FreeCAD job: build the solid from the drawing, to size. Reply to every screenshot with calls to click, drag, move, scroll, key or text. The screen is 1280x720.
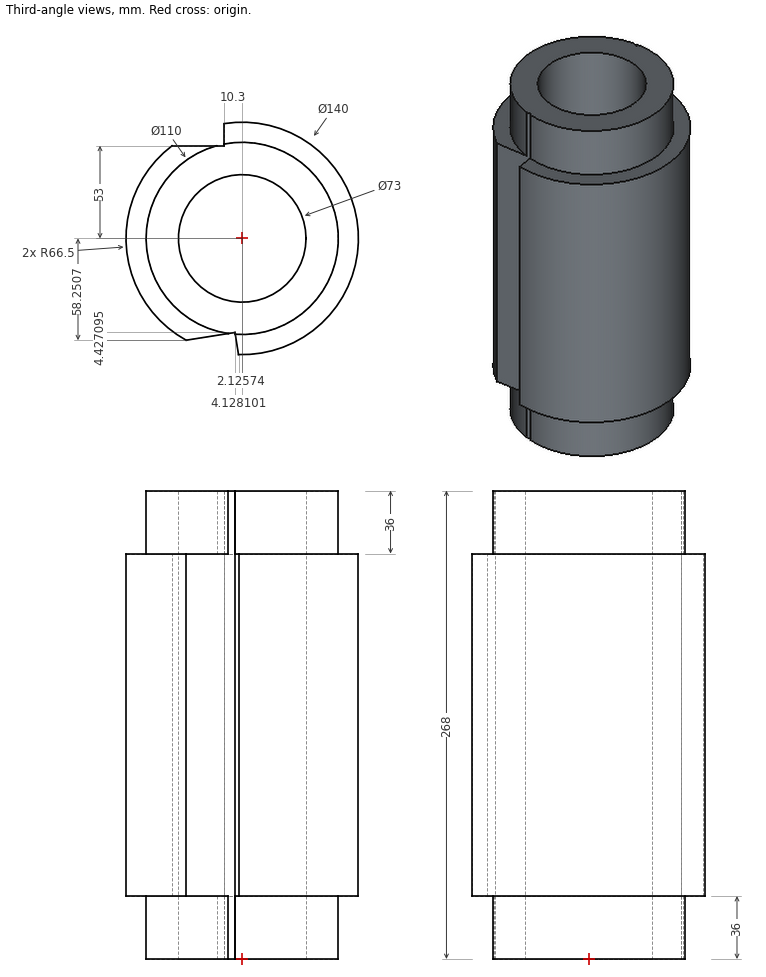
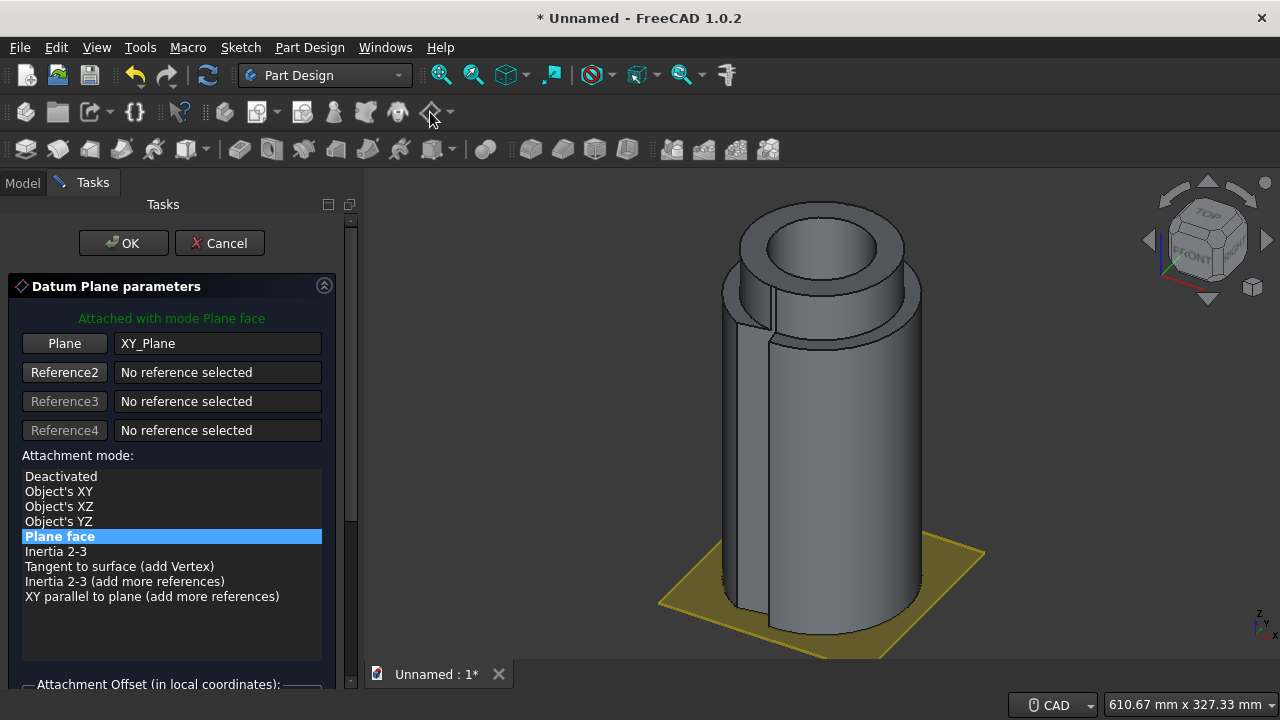
scroll(351, 451, down, 3)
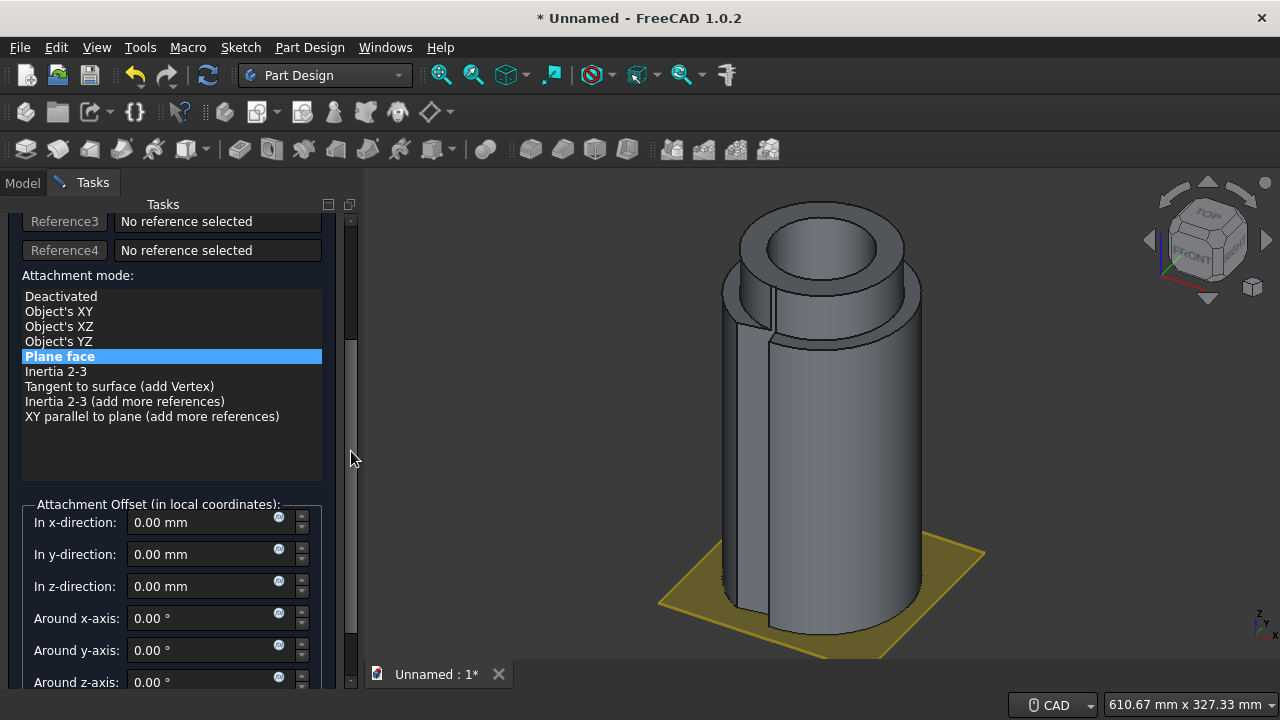
triple_click(210, 586)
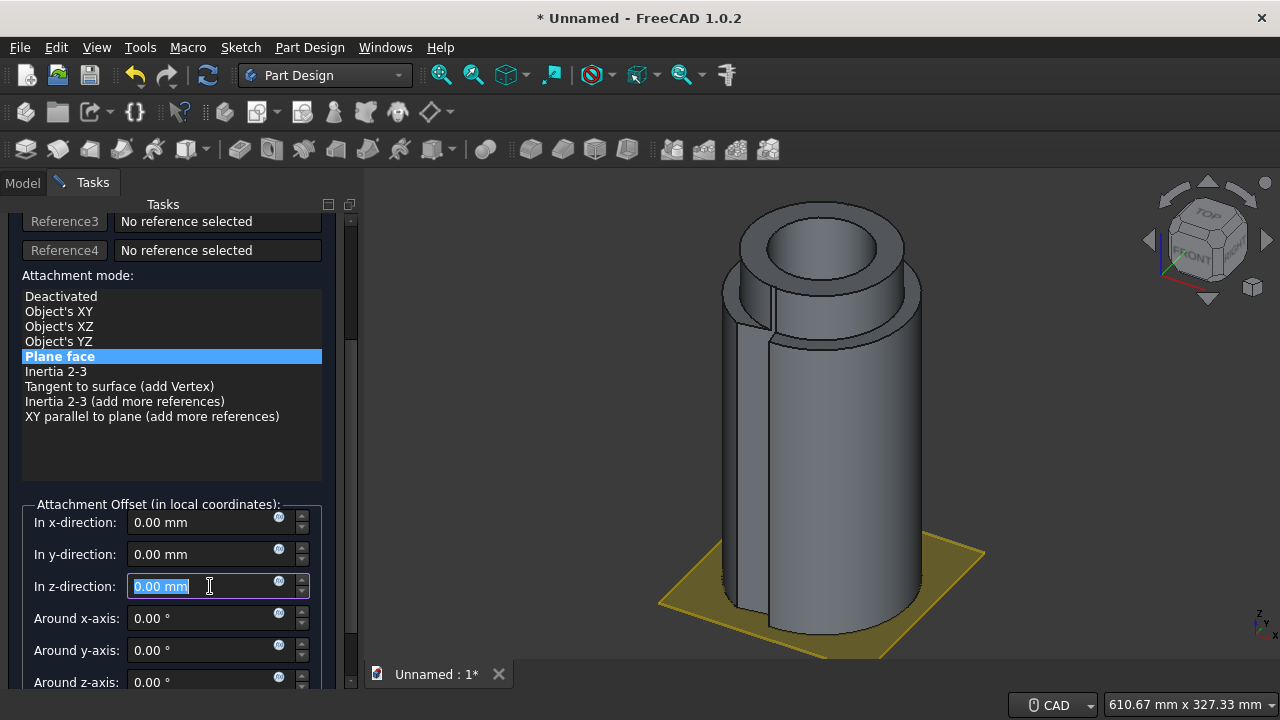
text(36)
key(Tab)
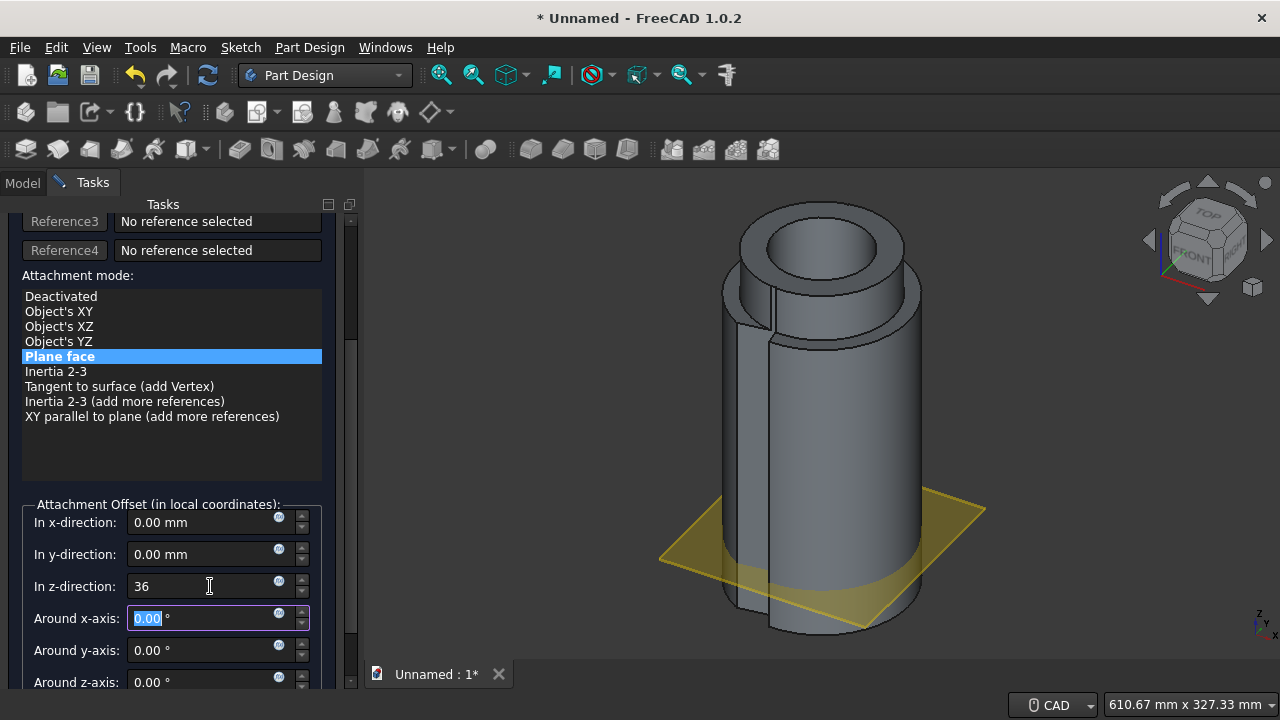
scroll(351, 451, up, 4)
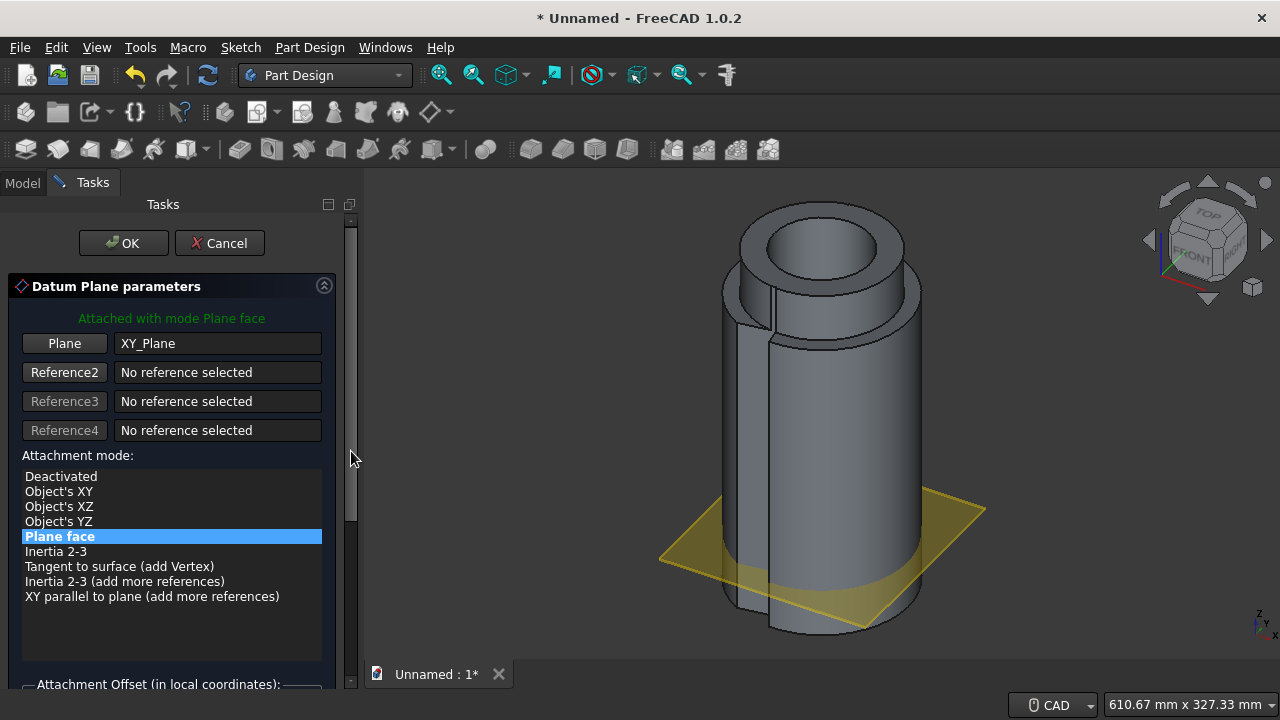
click(124, 243)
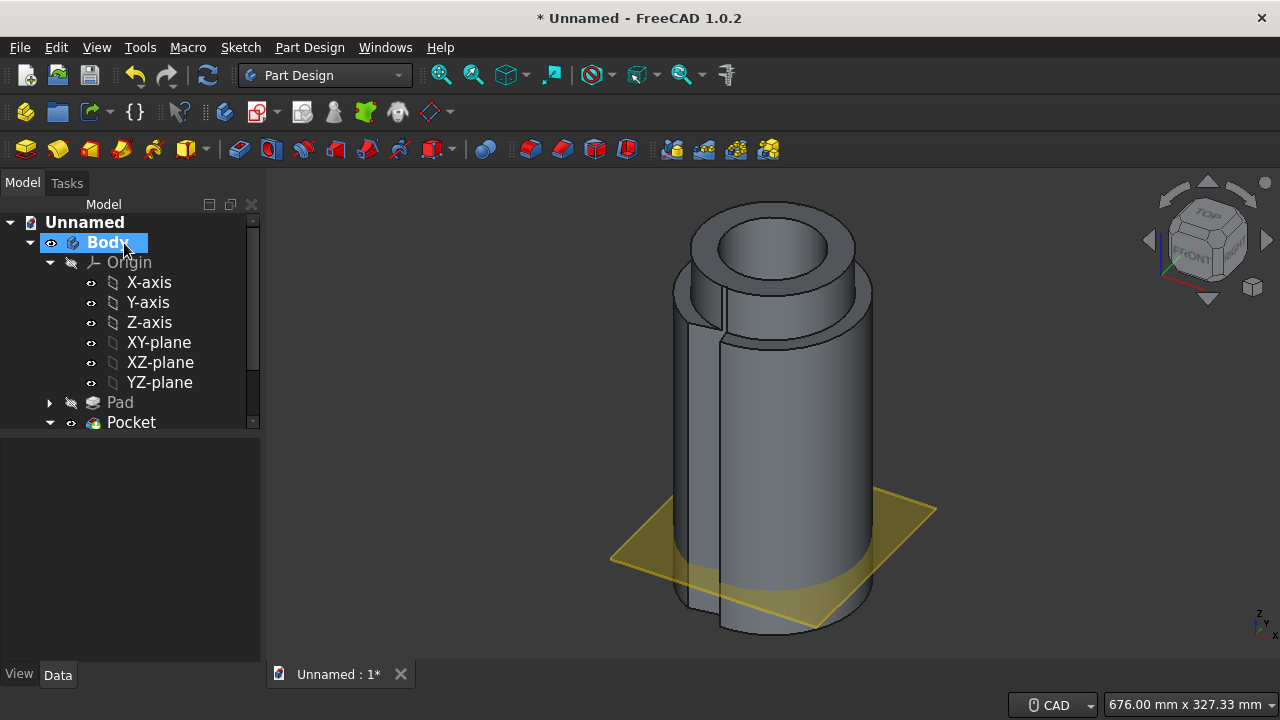
scroll(100, 318, down, 3)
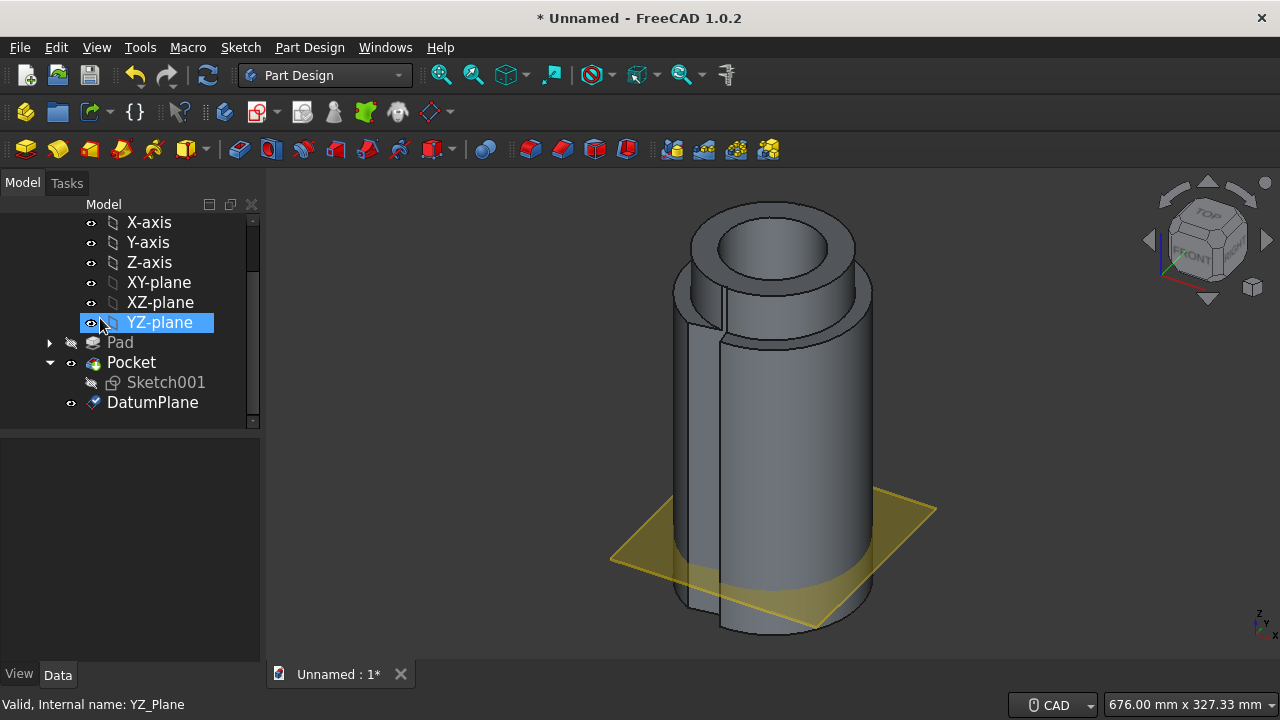
click(116, 403)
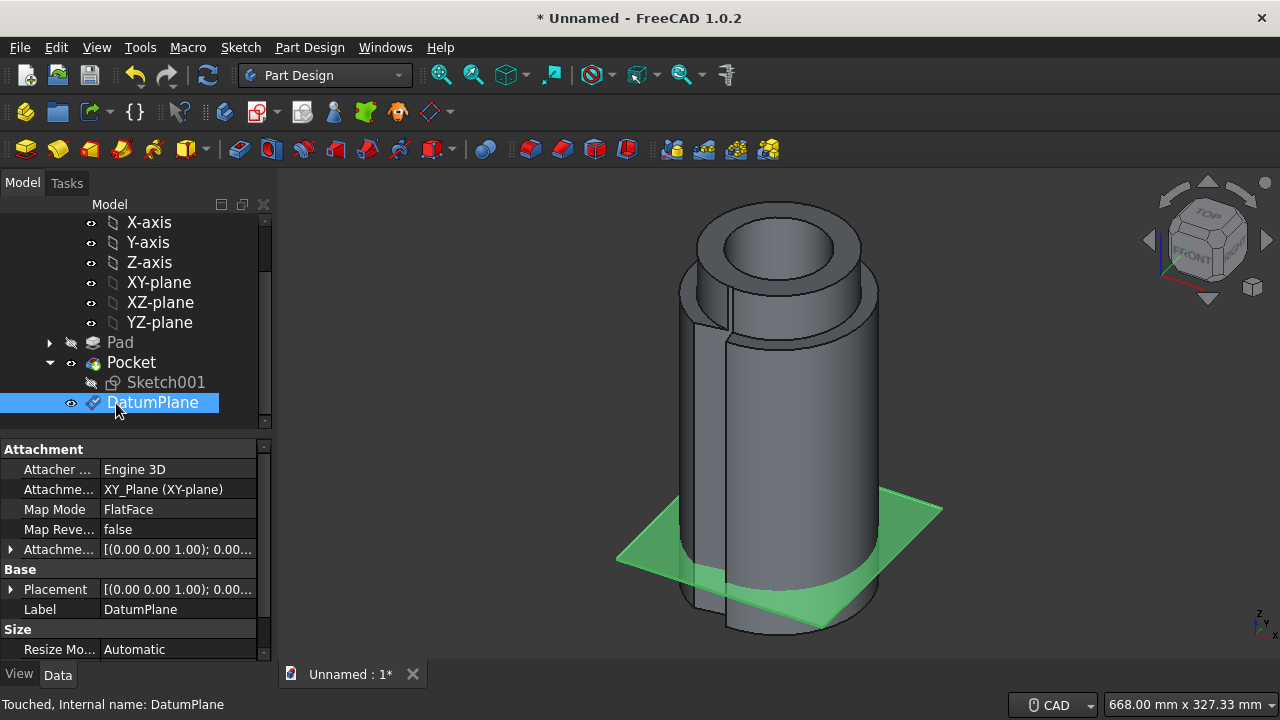
click(258, 112)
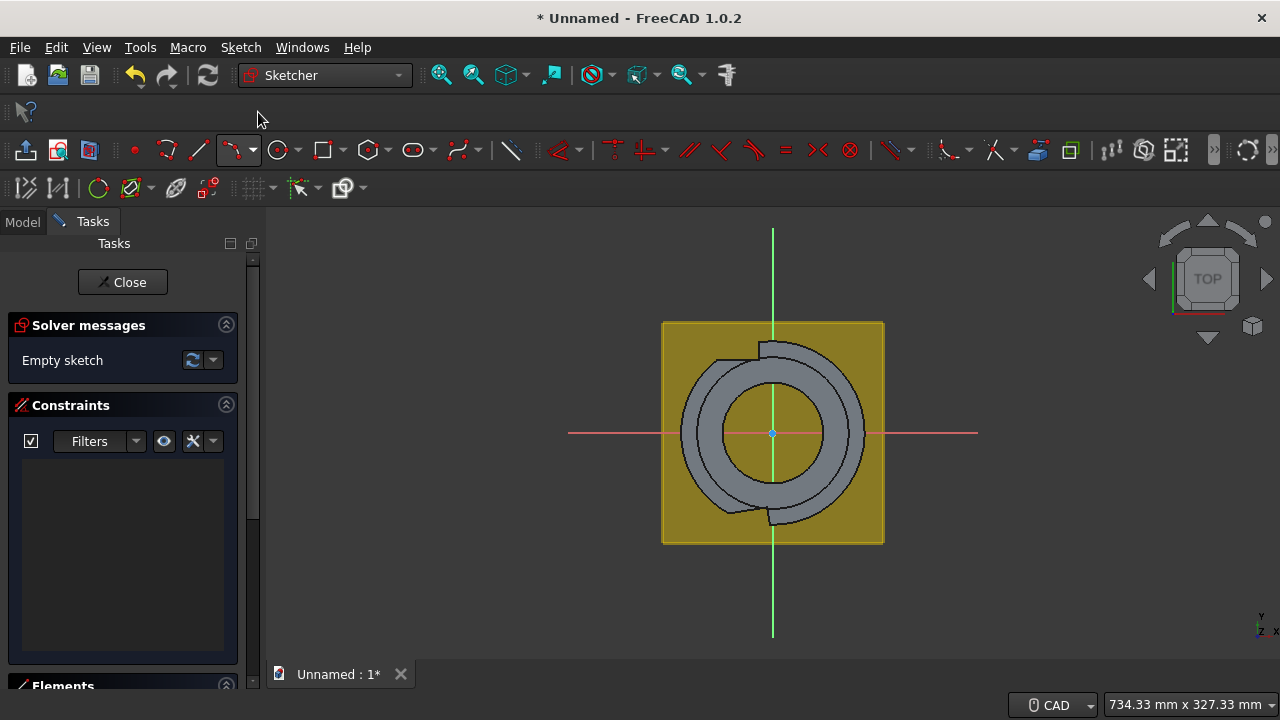
click(90, 150)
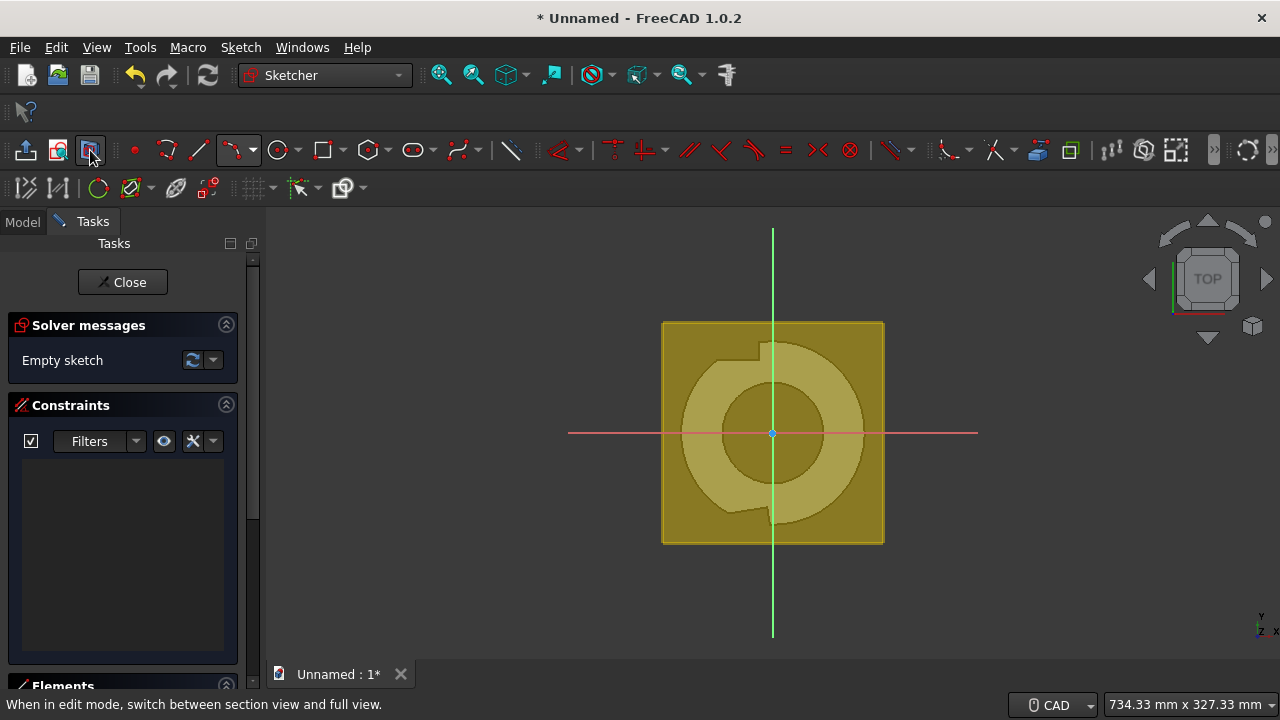
scroll(912, 433, up, 2)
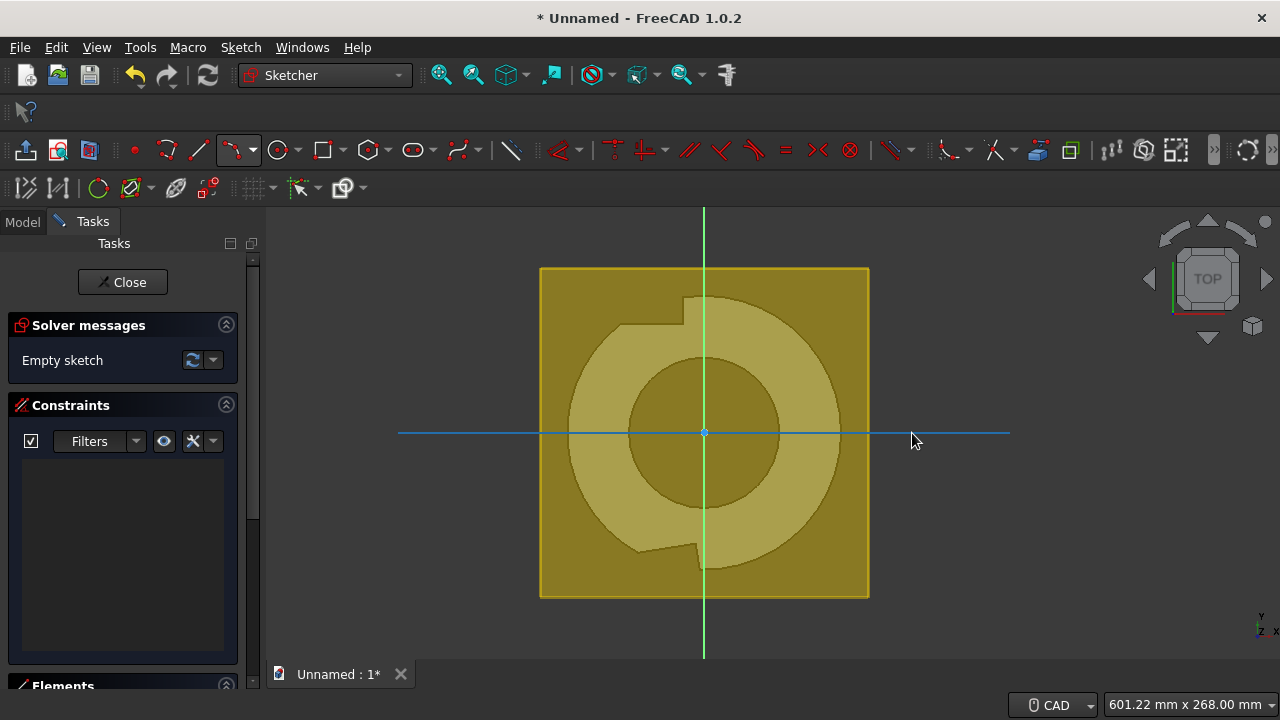
click(278, 150)